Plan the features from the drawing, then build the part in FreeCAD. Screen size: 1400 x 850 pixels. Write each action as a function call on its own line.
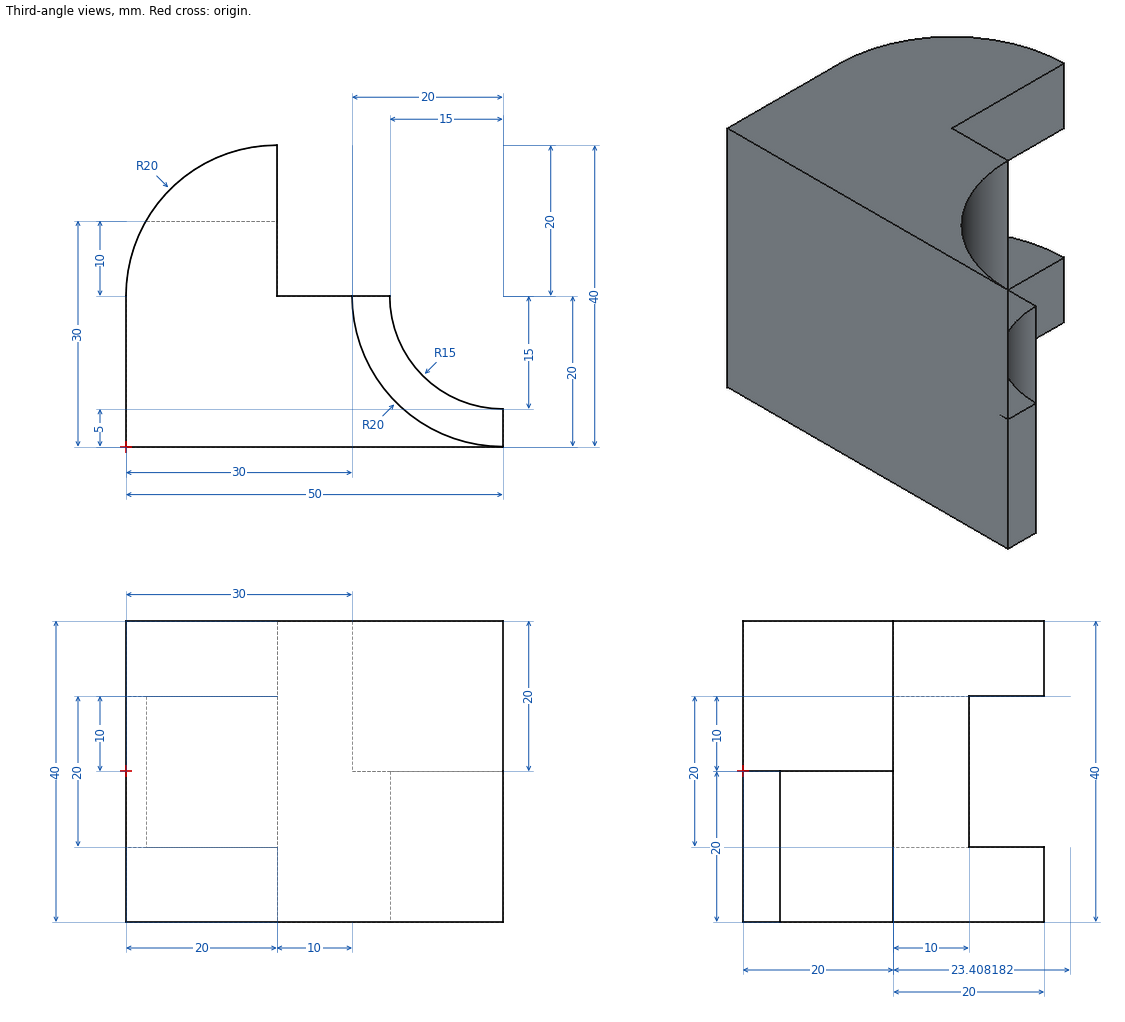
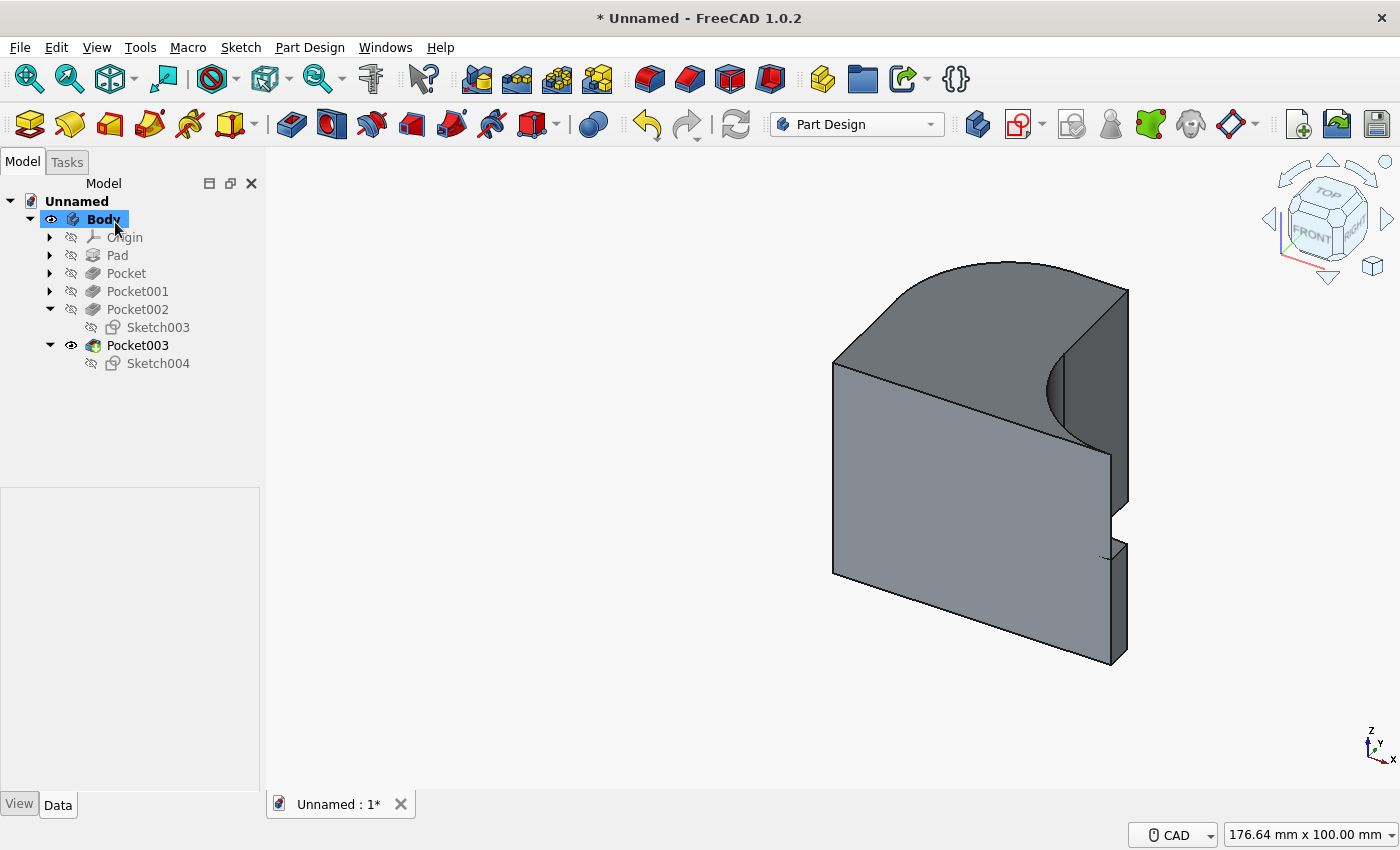
key(6)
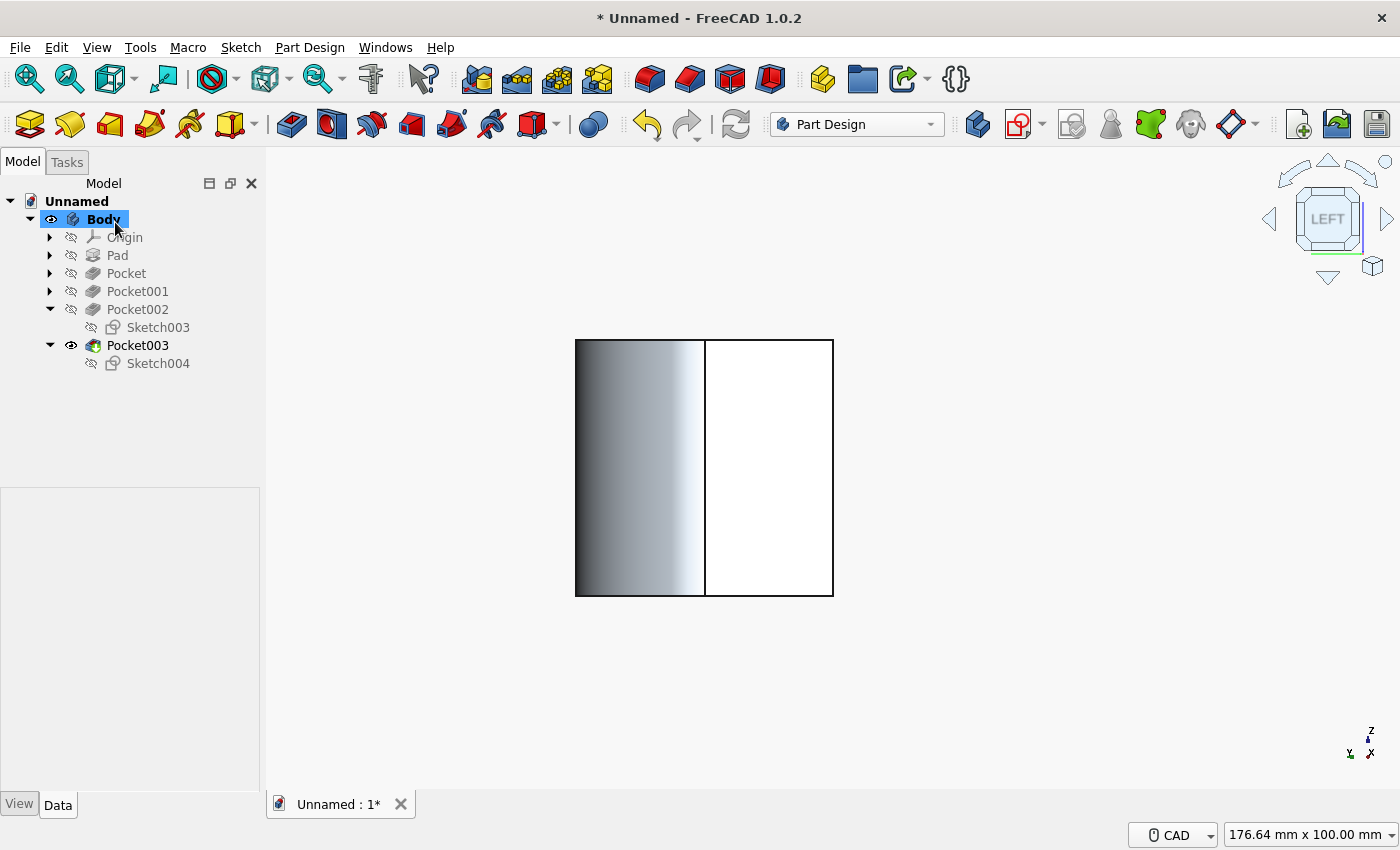
key(v)
key(f)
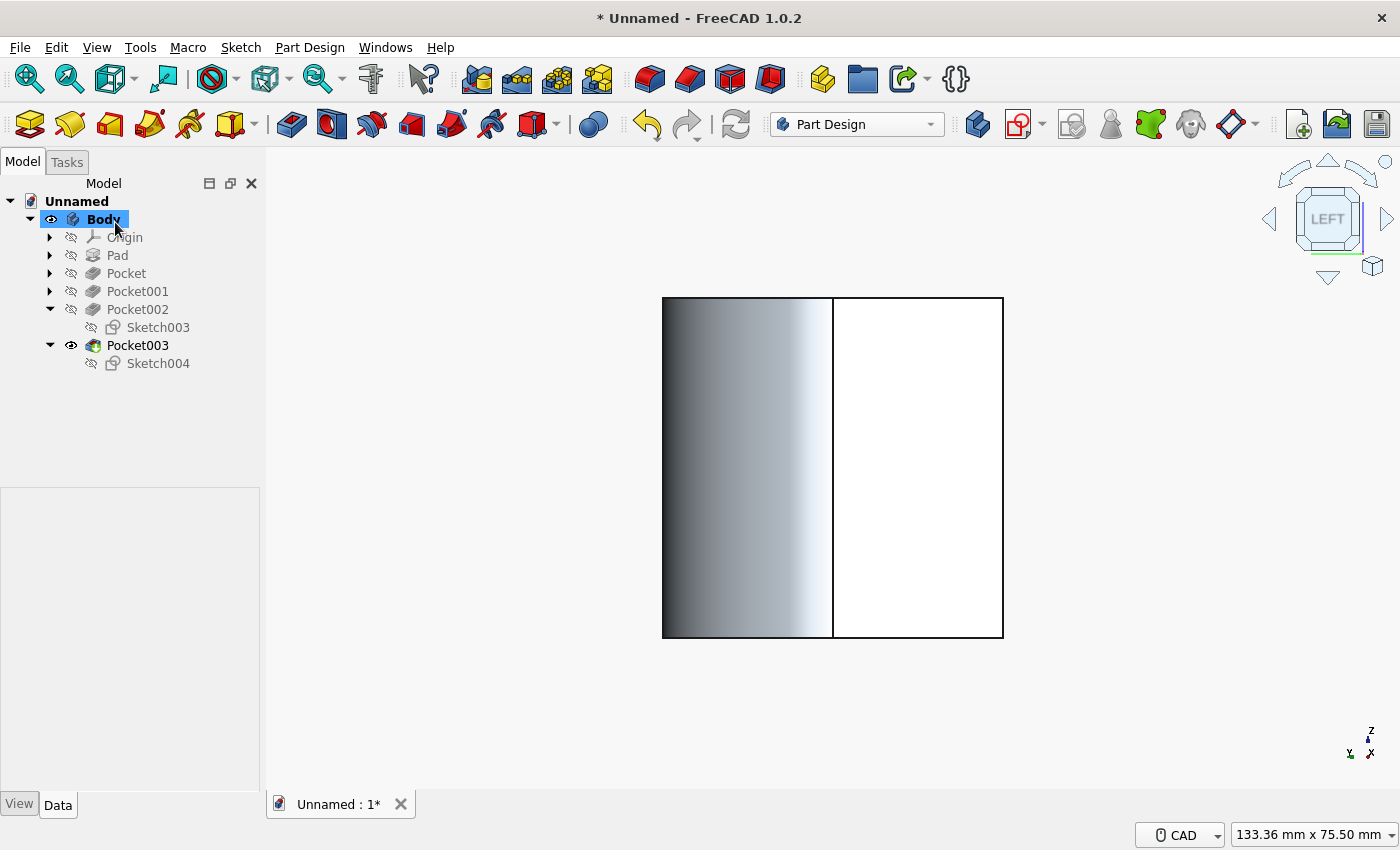
click(918, 418)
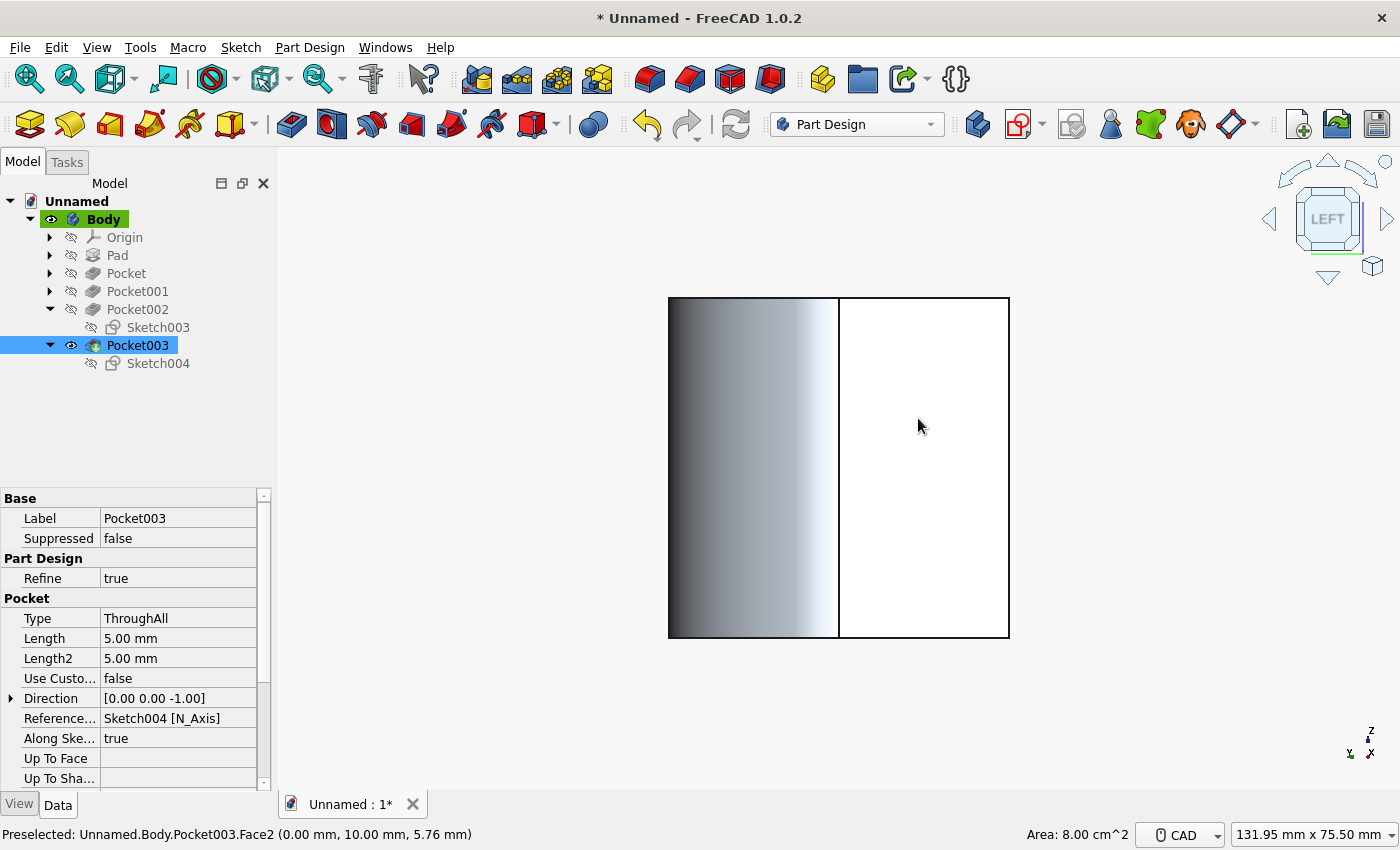
click(1018, 124)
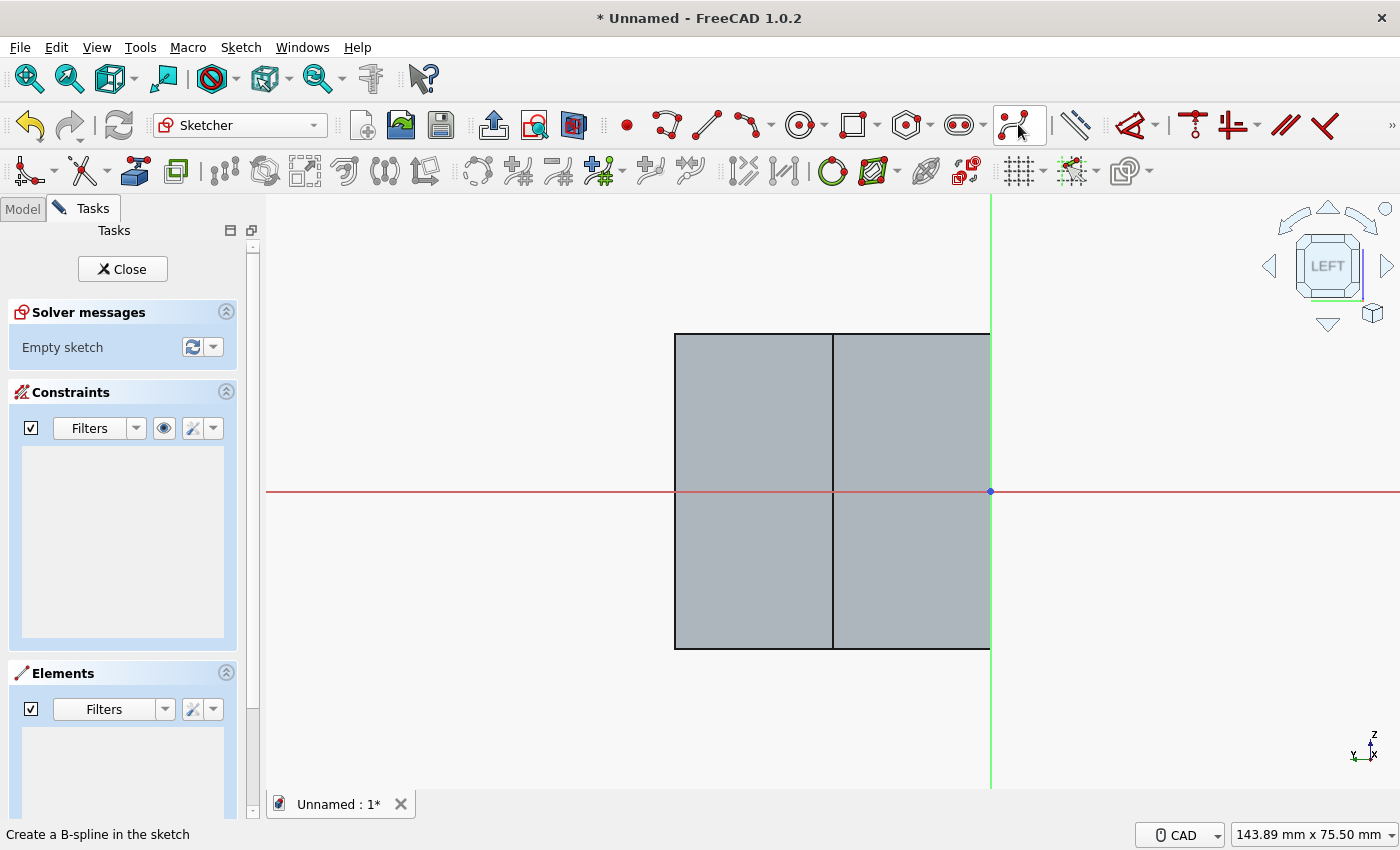
scroll(887, 492, up, 3)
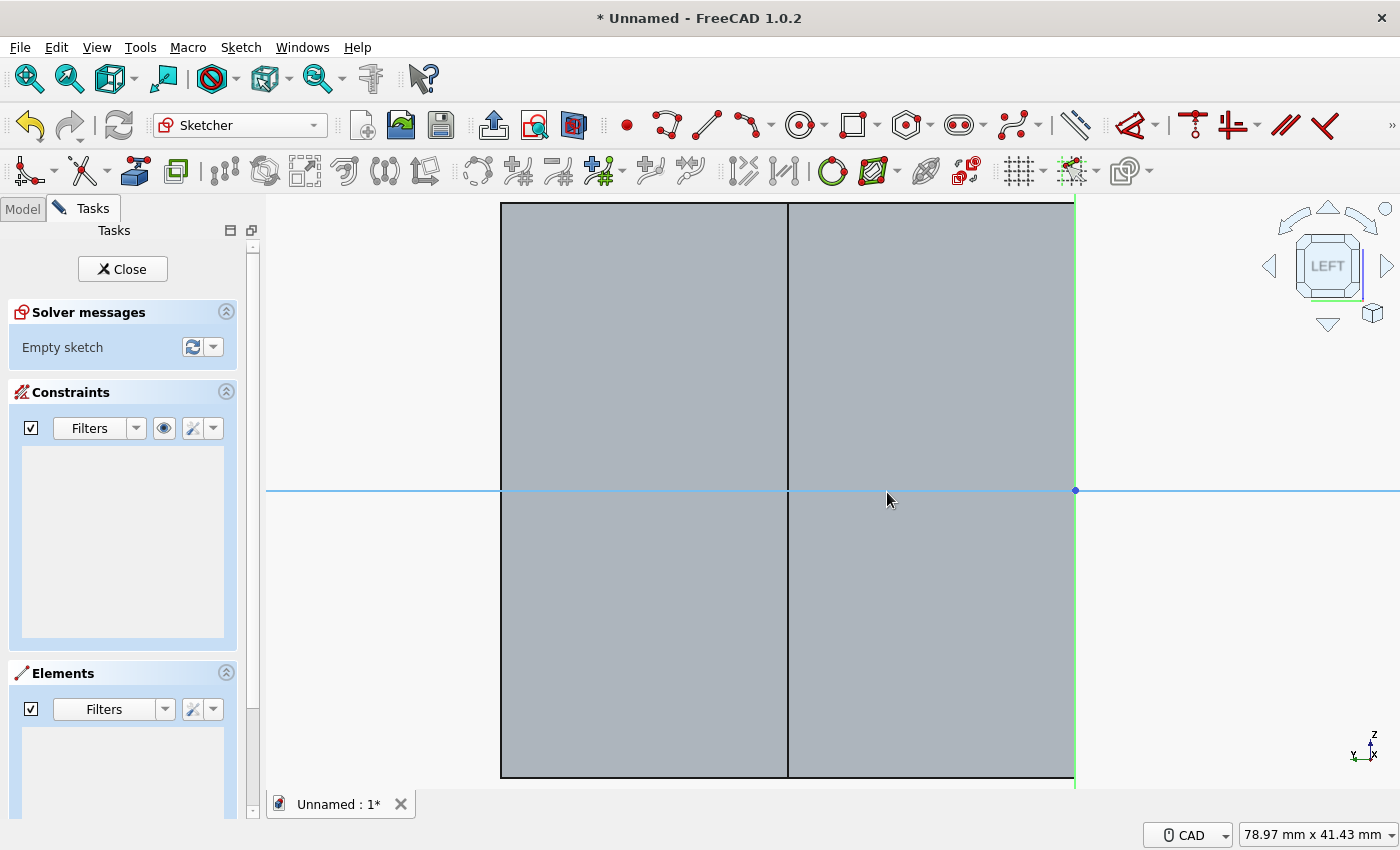
key(g)
key(r)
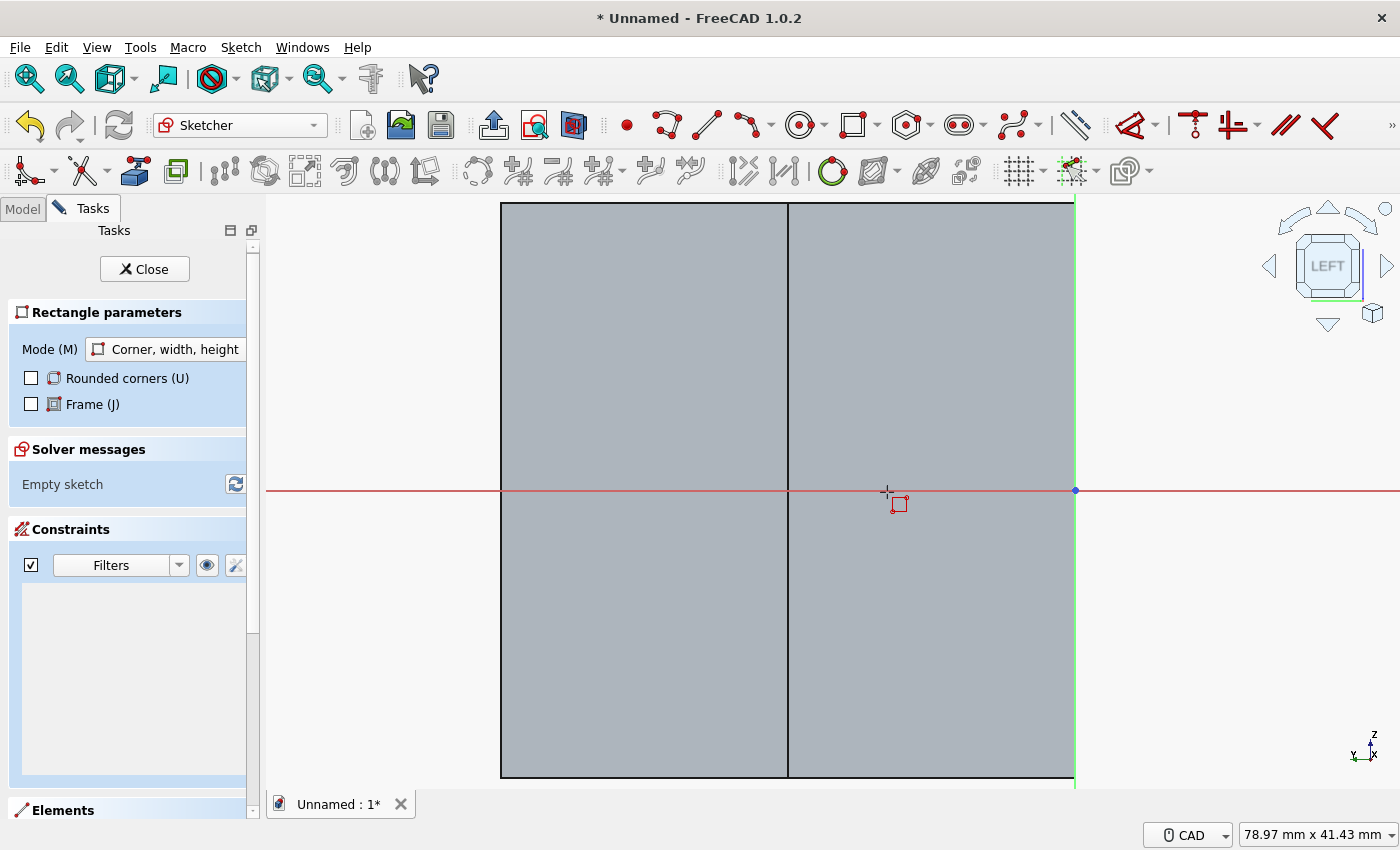
click(452, 347)
move(788, 634)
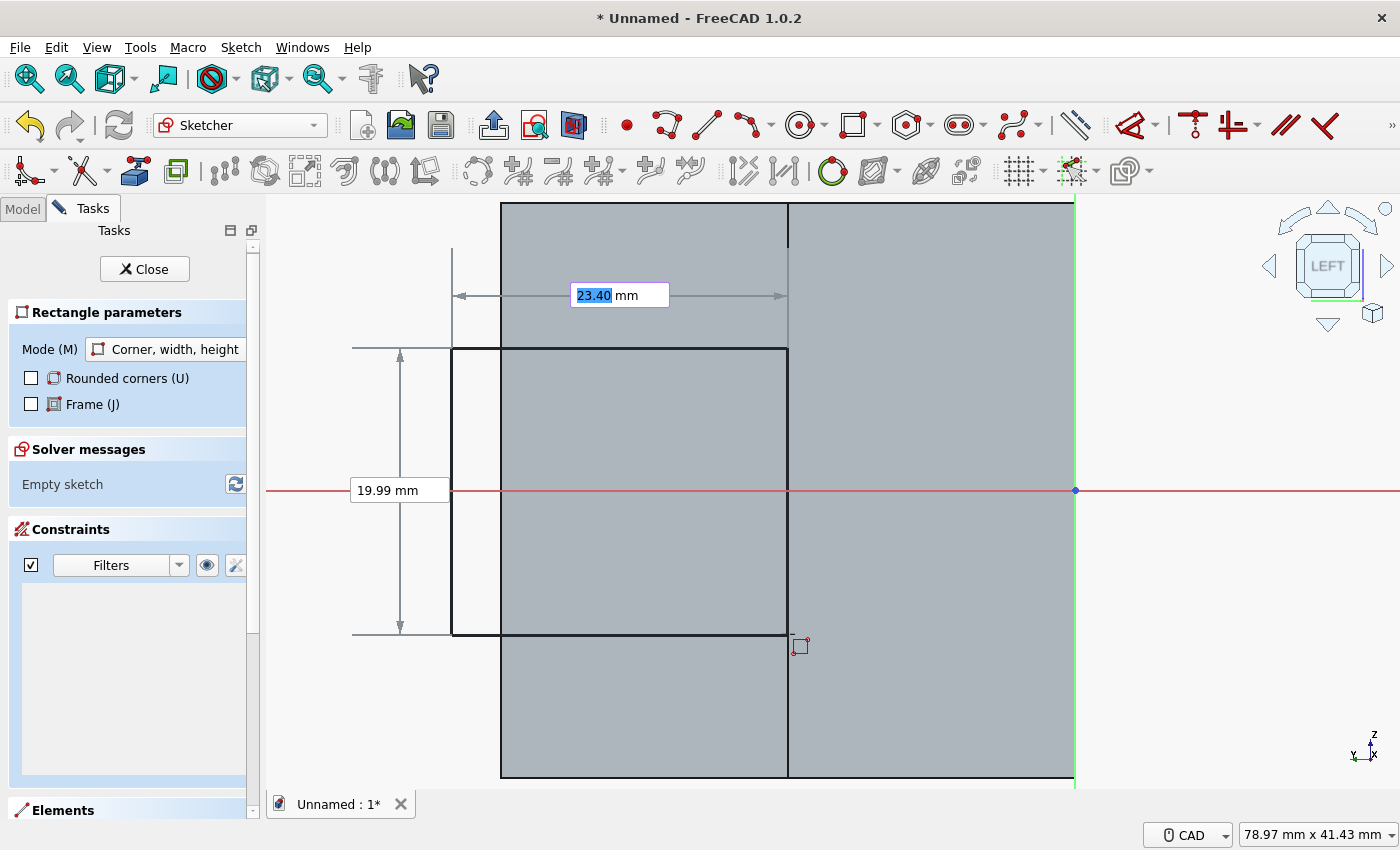
text(23.408182)
key(Tab)
text(20)
key(Return)
key(Escape)